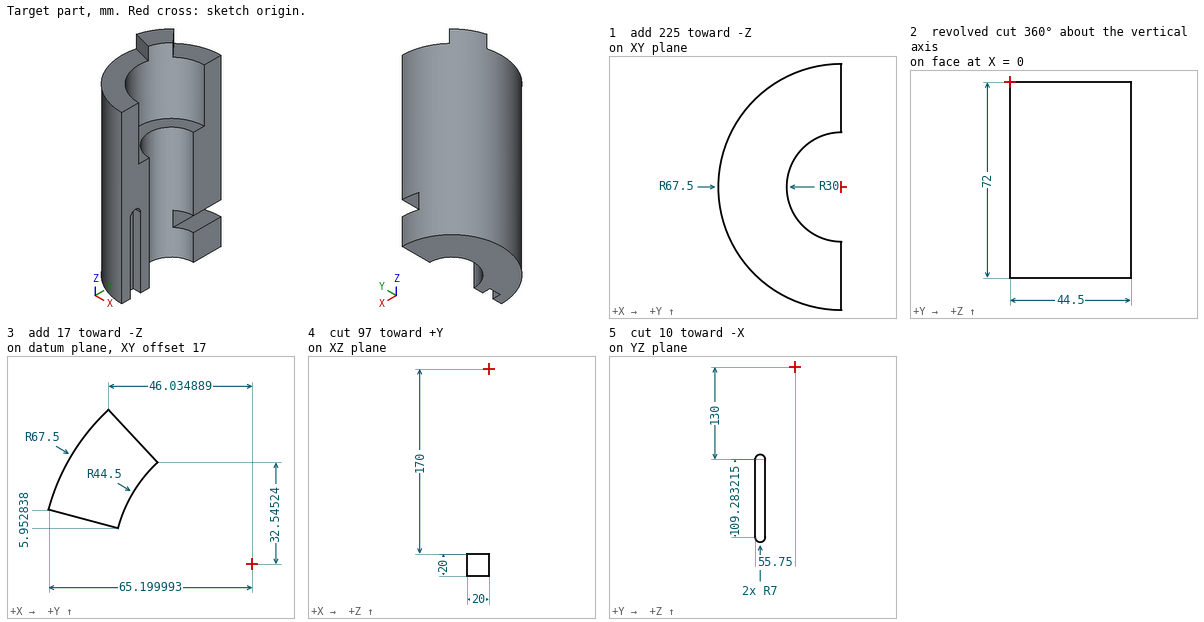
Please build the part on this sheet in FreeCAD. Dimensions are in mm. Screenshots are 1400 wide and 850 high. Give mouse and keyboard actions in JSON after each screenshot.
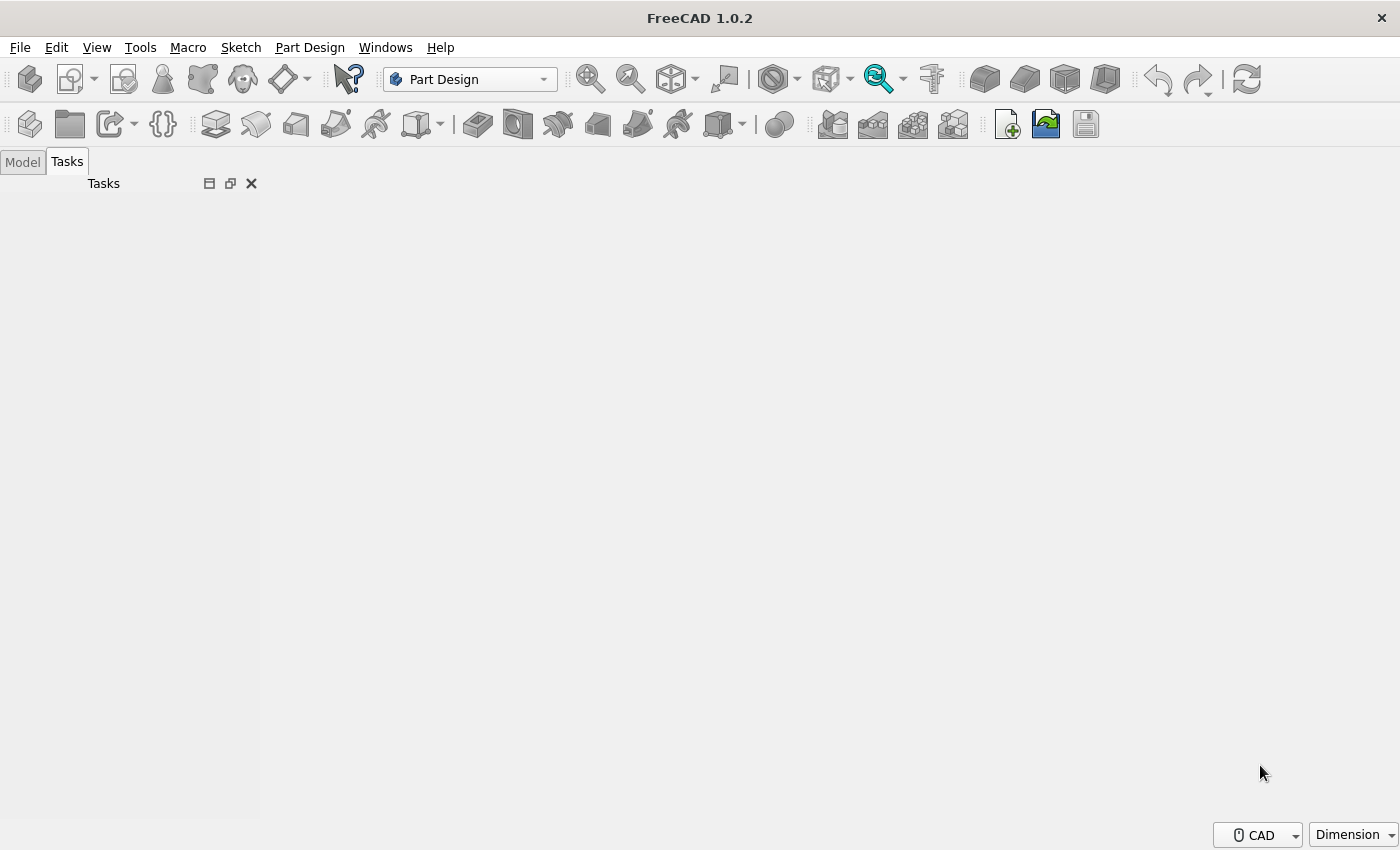
{"action": "key", "text": "ctrl+n"}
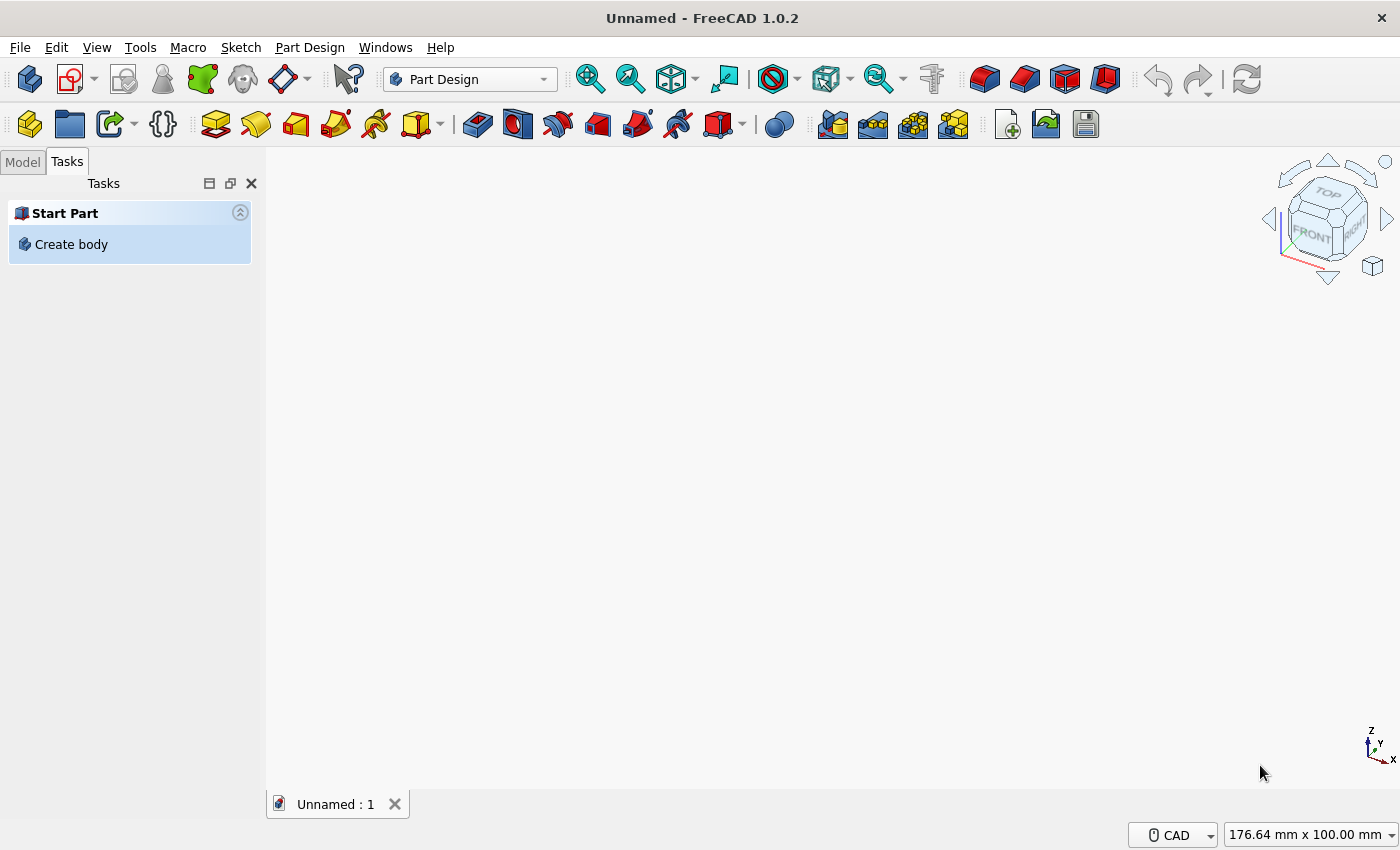
{"action": "left_click", "coordinate": [70, 80]}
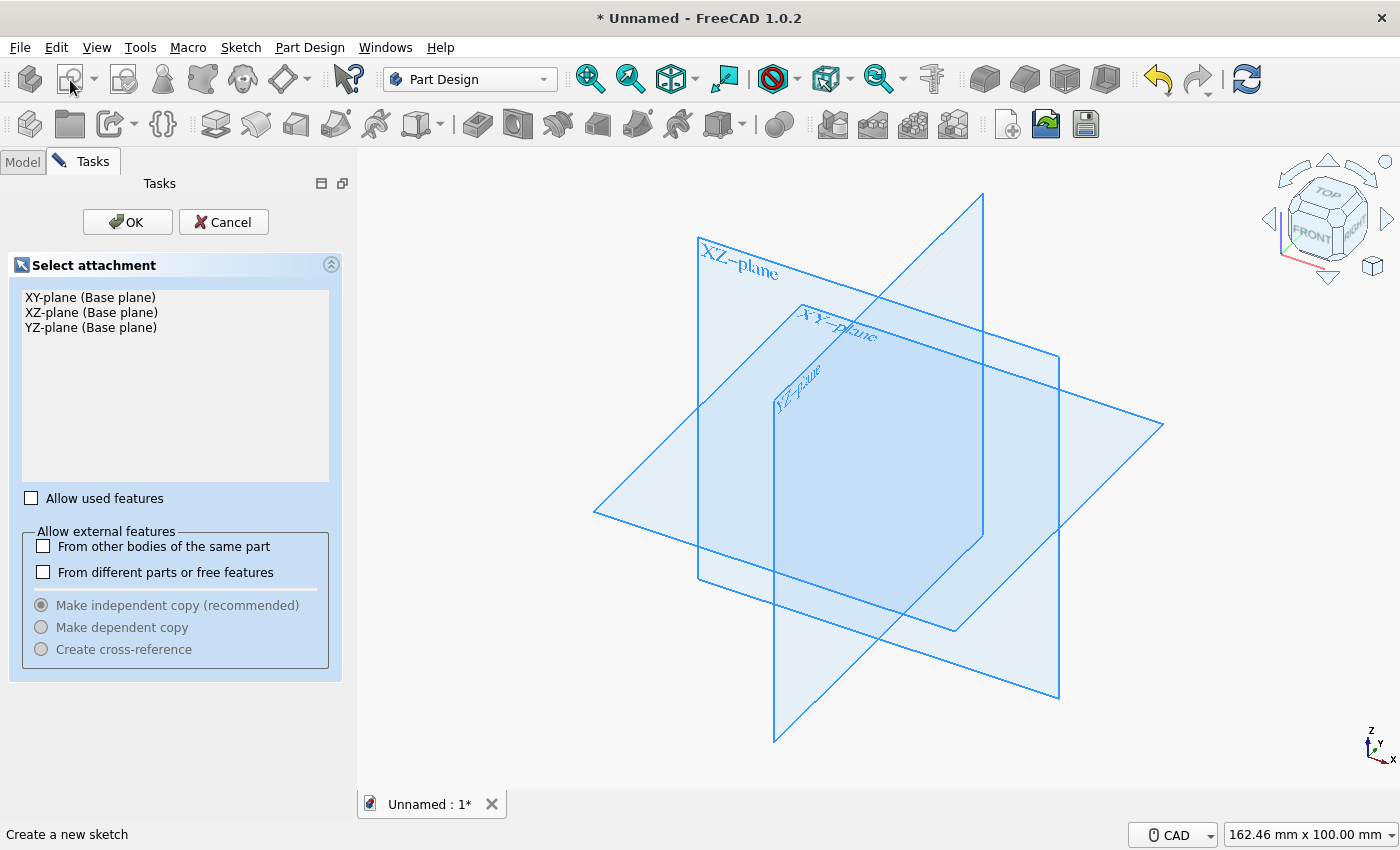
{"action": "left_click", "coordinate": [82, 298]}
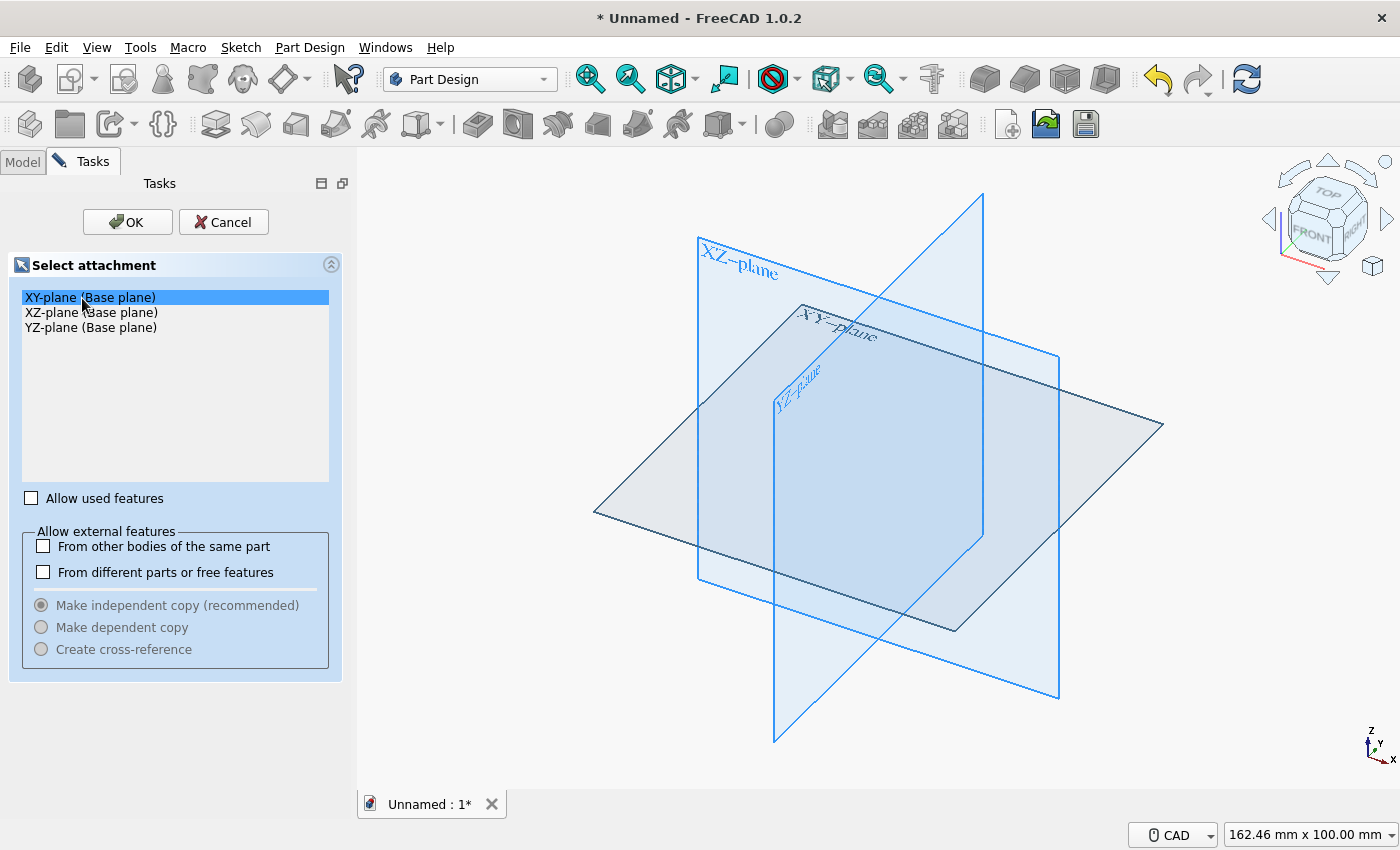
{"action": "left_click", "coordinate": [128, 222]}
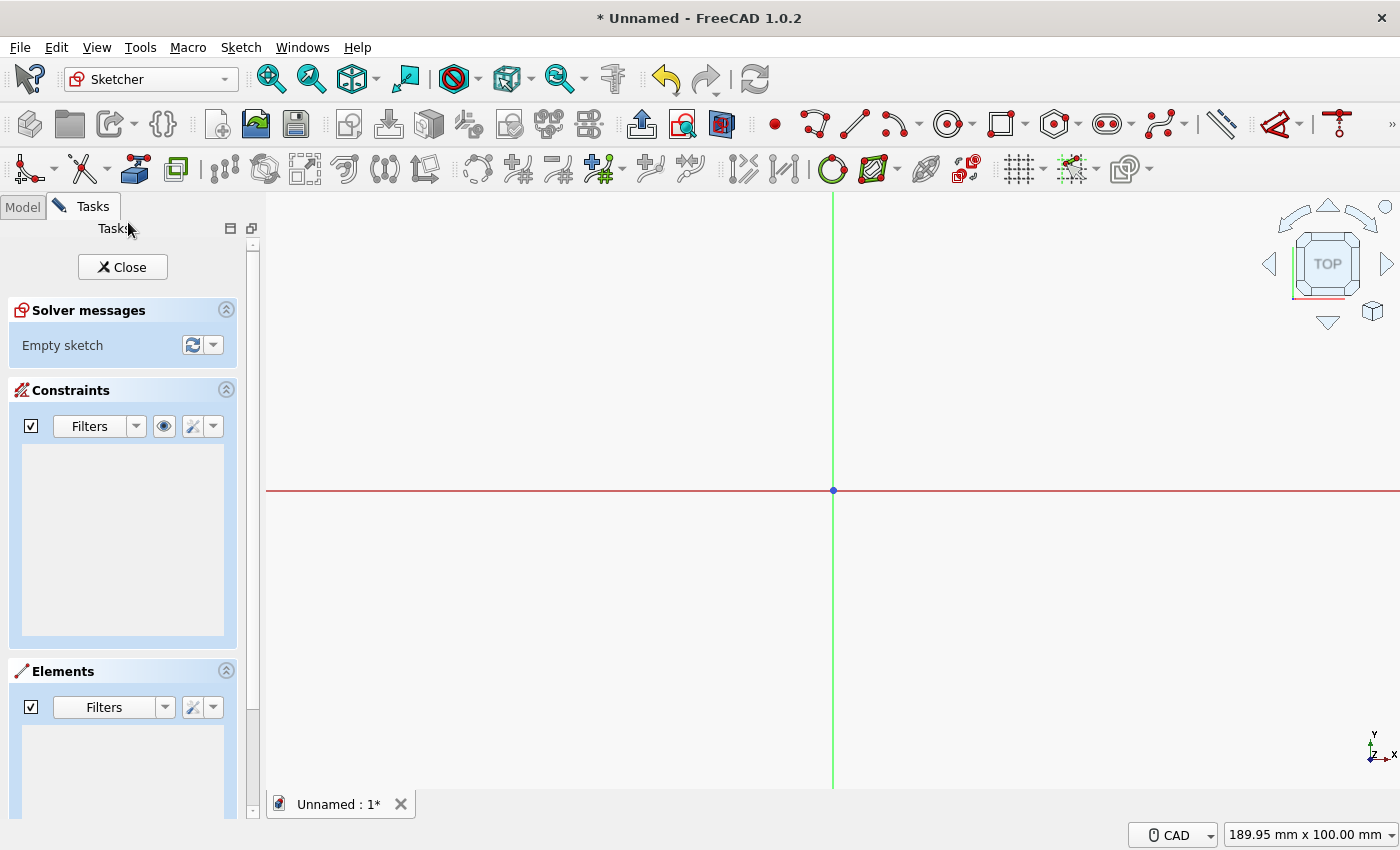
{"action": "scroll", "coordinate": [873, 490], "scroll_direction": "down", "scroll_amount": 4}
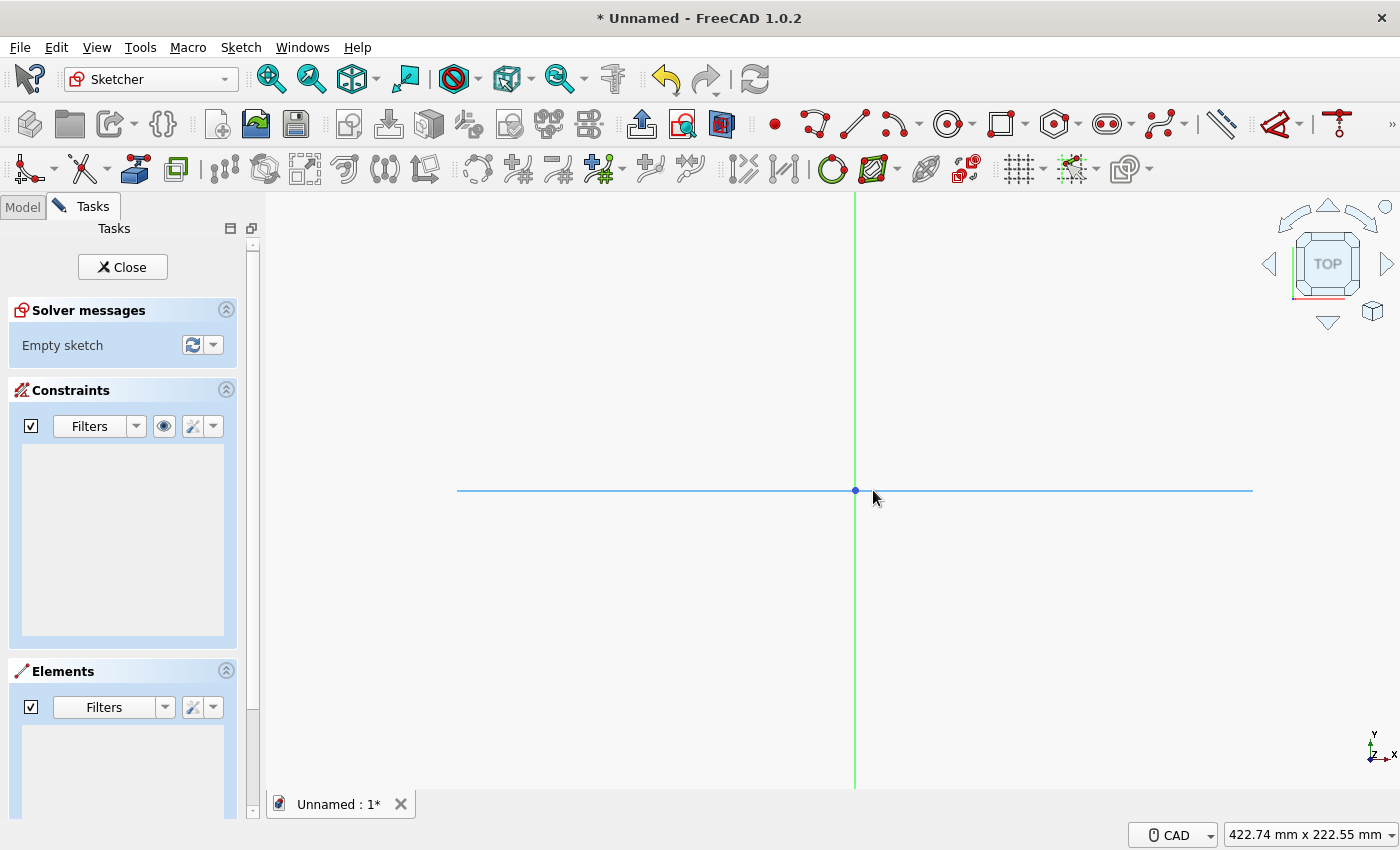
{"action": "left_click", "coordinate": [856, 124]}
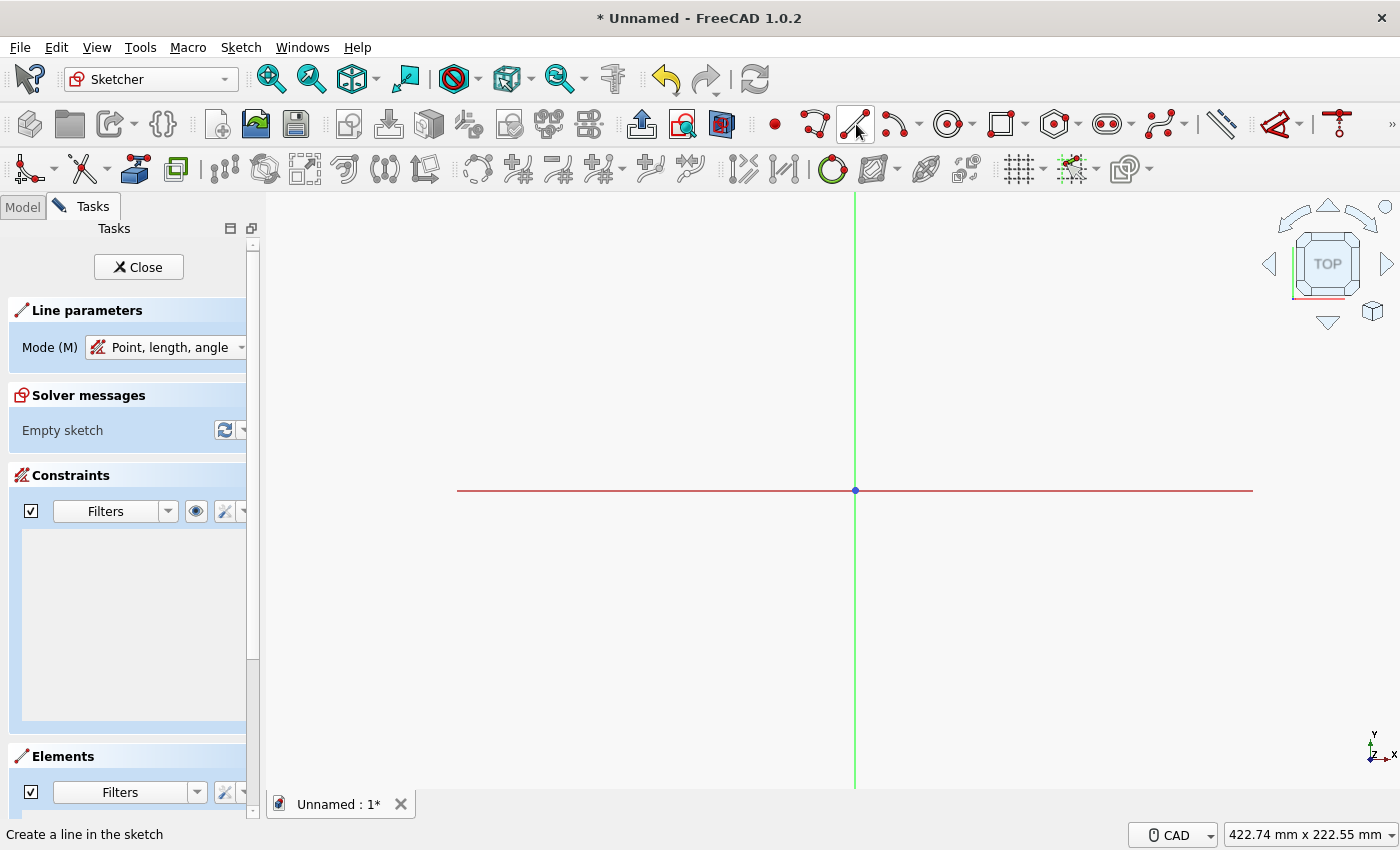
{"action": "left_click", "coordinate": [855, 410]}
{"action": "left_click", "coordinate": [846, 309]}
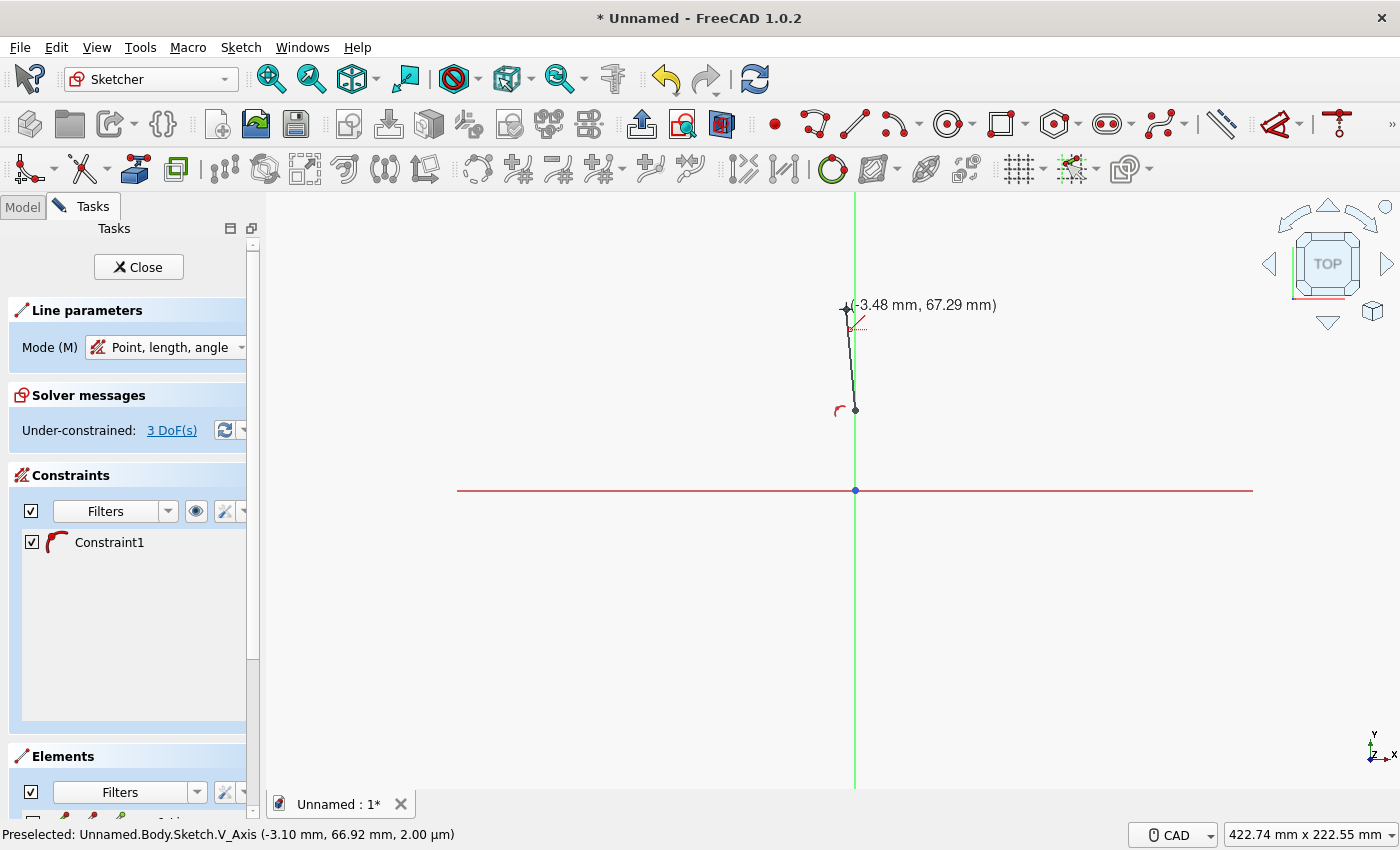
{"action": "left_click", "coordinate": [855, 672]}
{"action": "left_click", "coordinate": [846, 571]}